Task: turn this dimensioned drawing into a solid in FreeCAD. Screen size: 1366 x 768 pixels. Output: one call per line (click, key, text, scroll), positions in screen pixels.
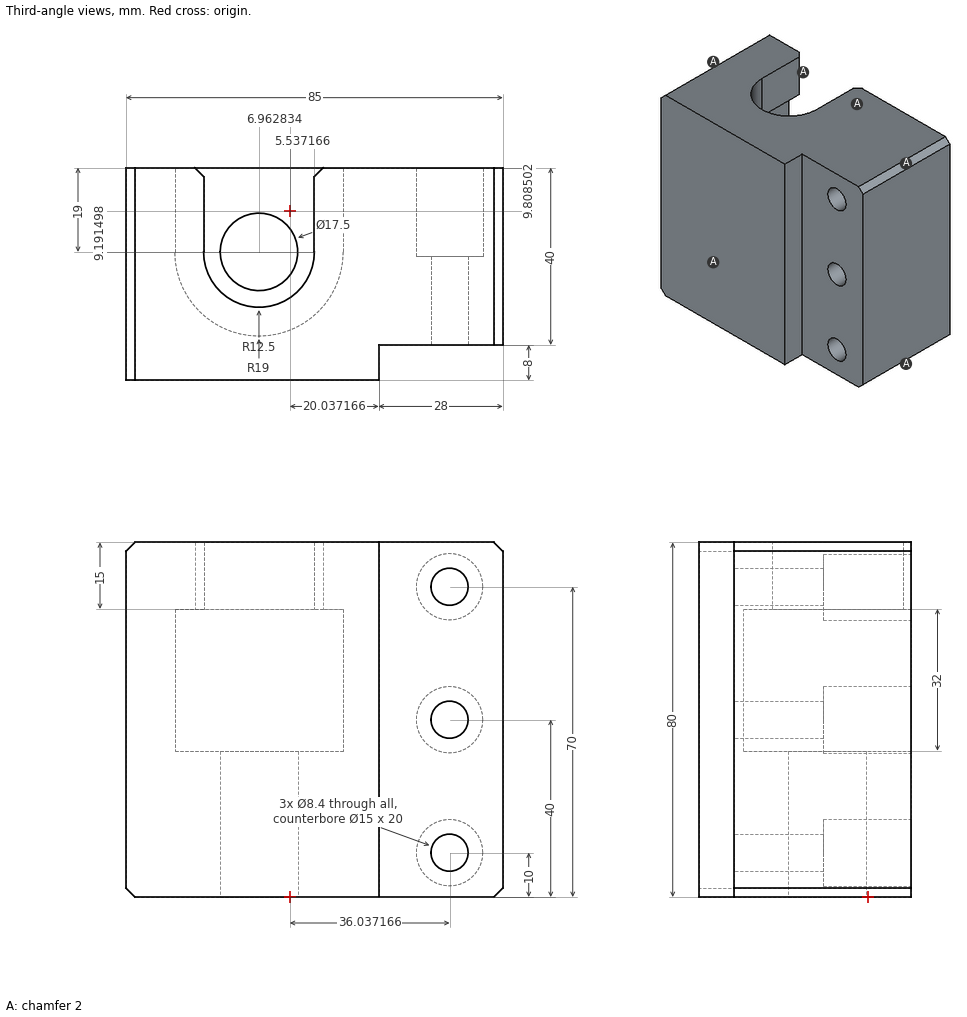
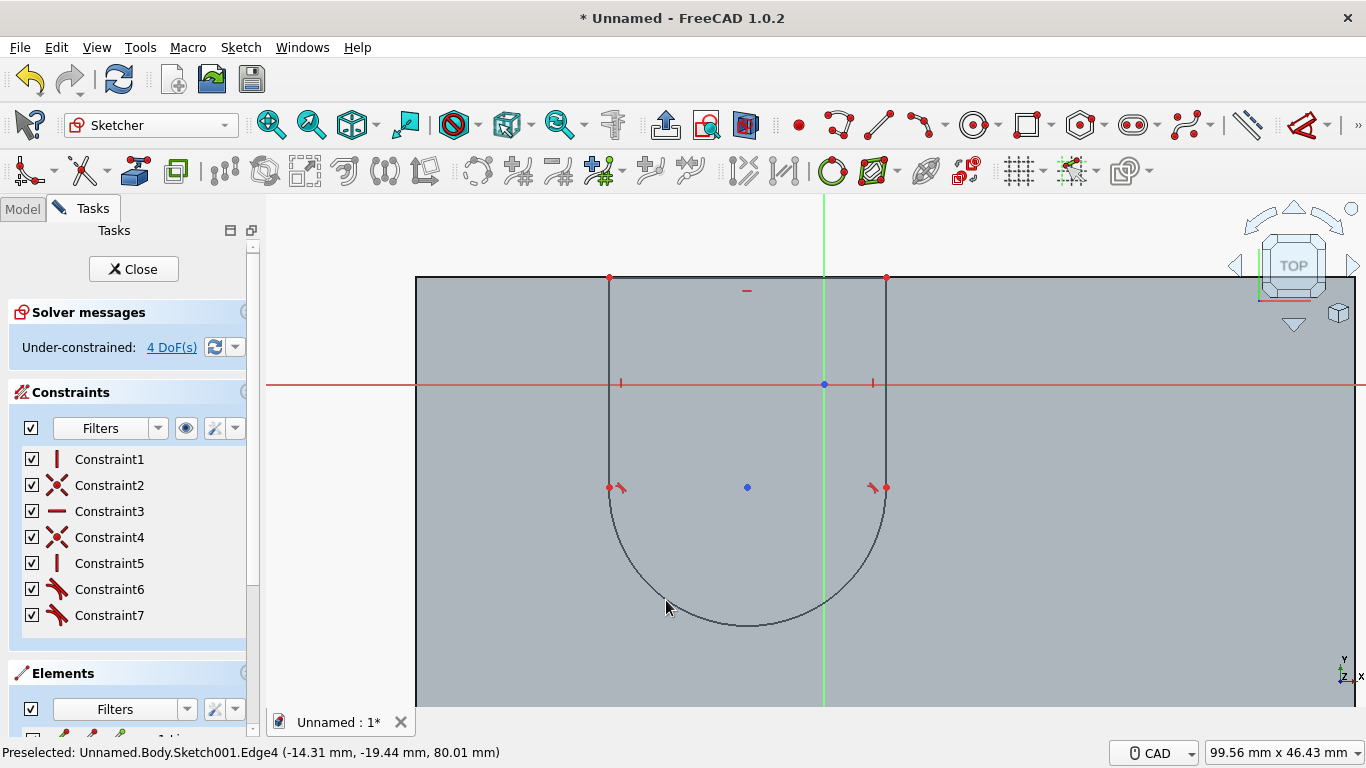
click(1302, 126)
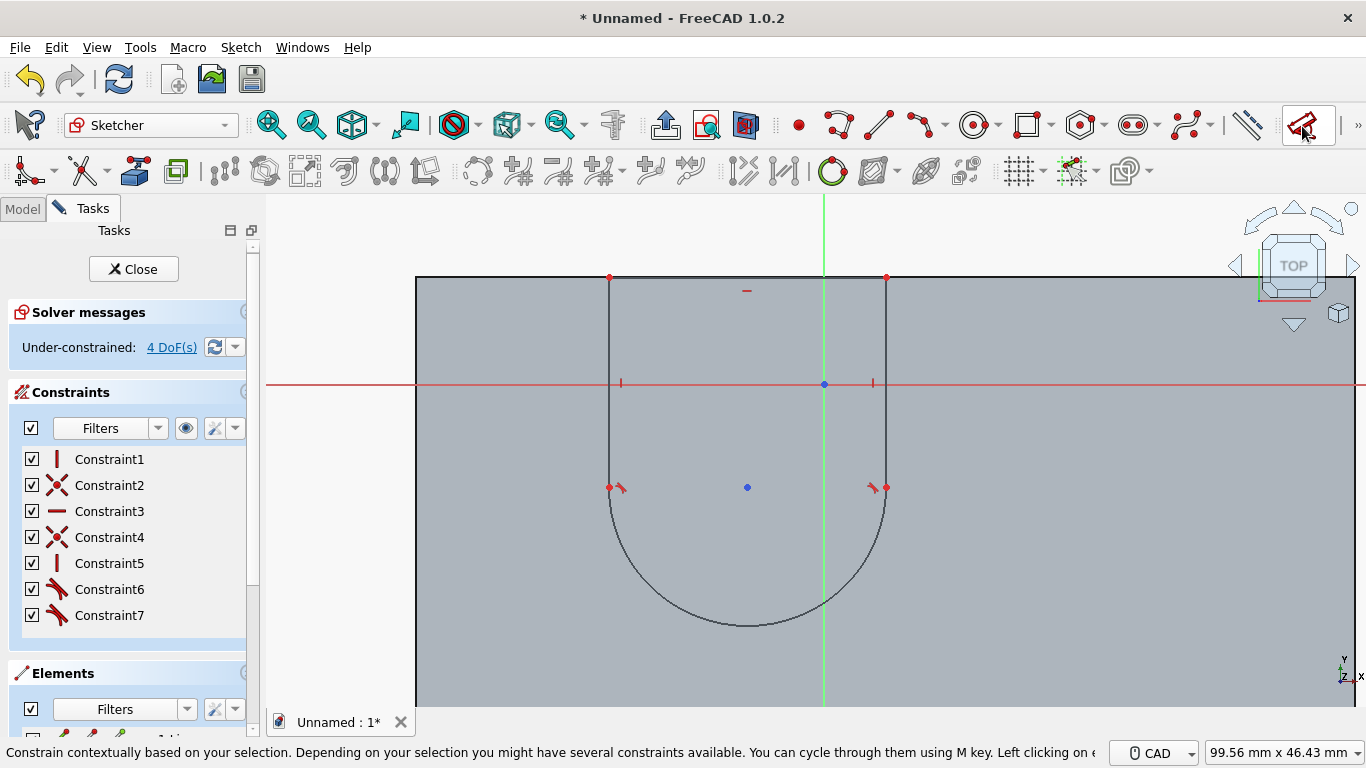
click(666, 600)
click(647, 626)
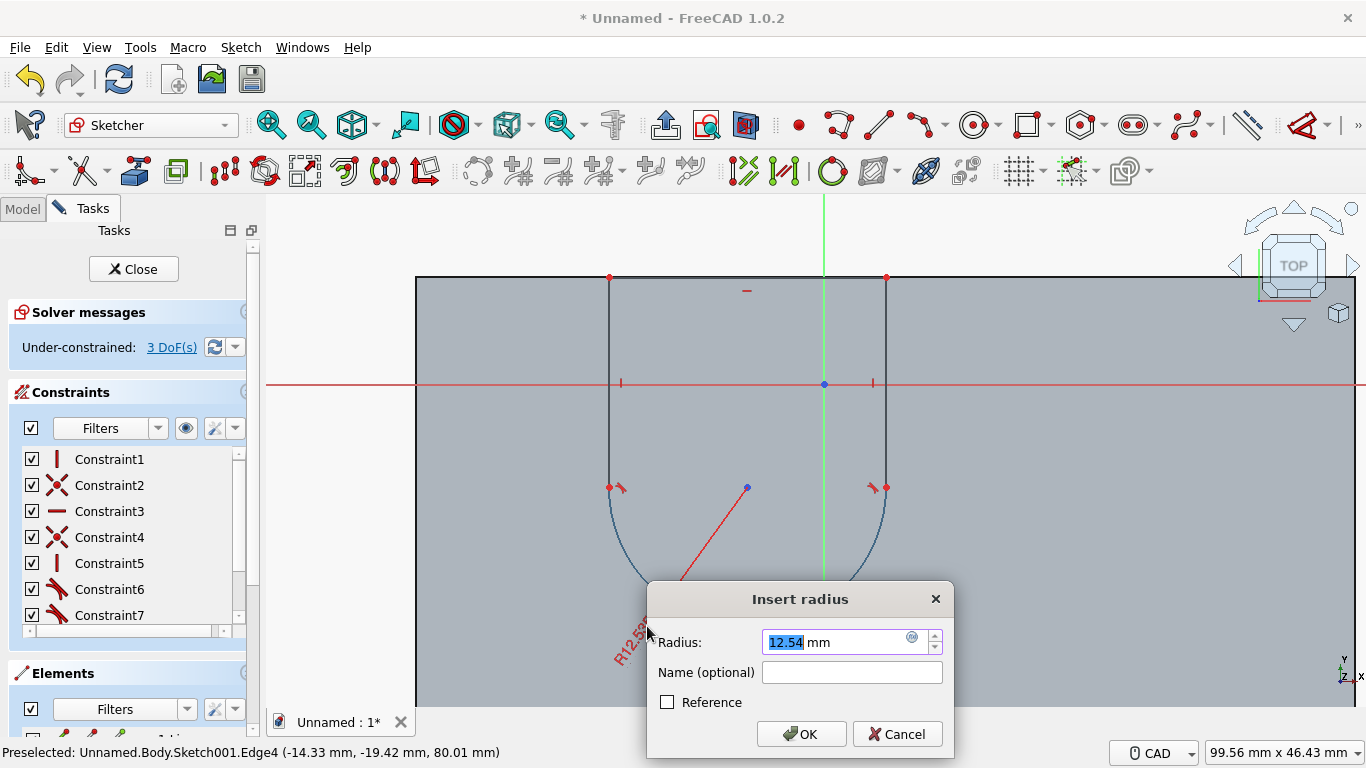
text(12.5)
key(Return)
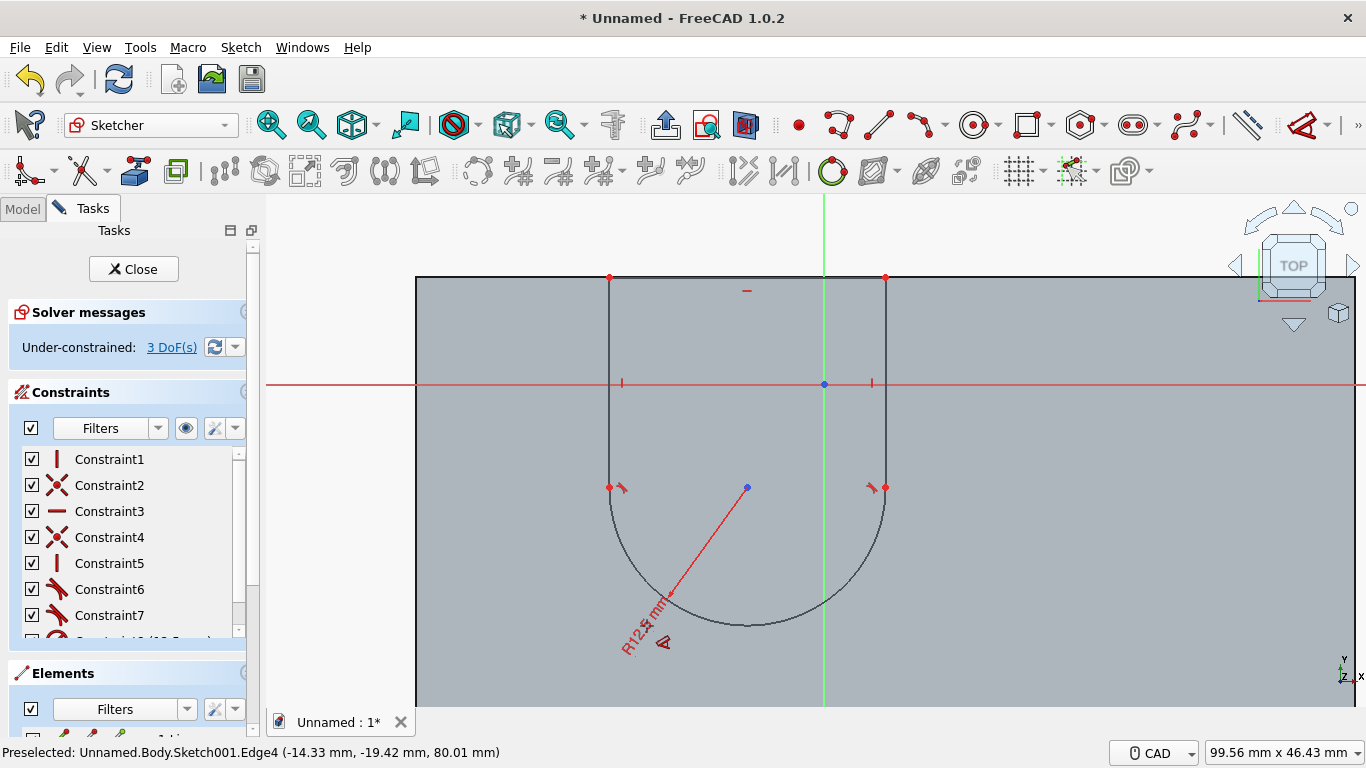
click(886, 425)
click(920, 335)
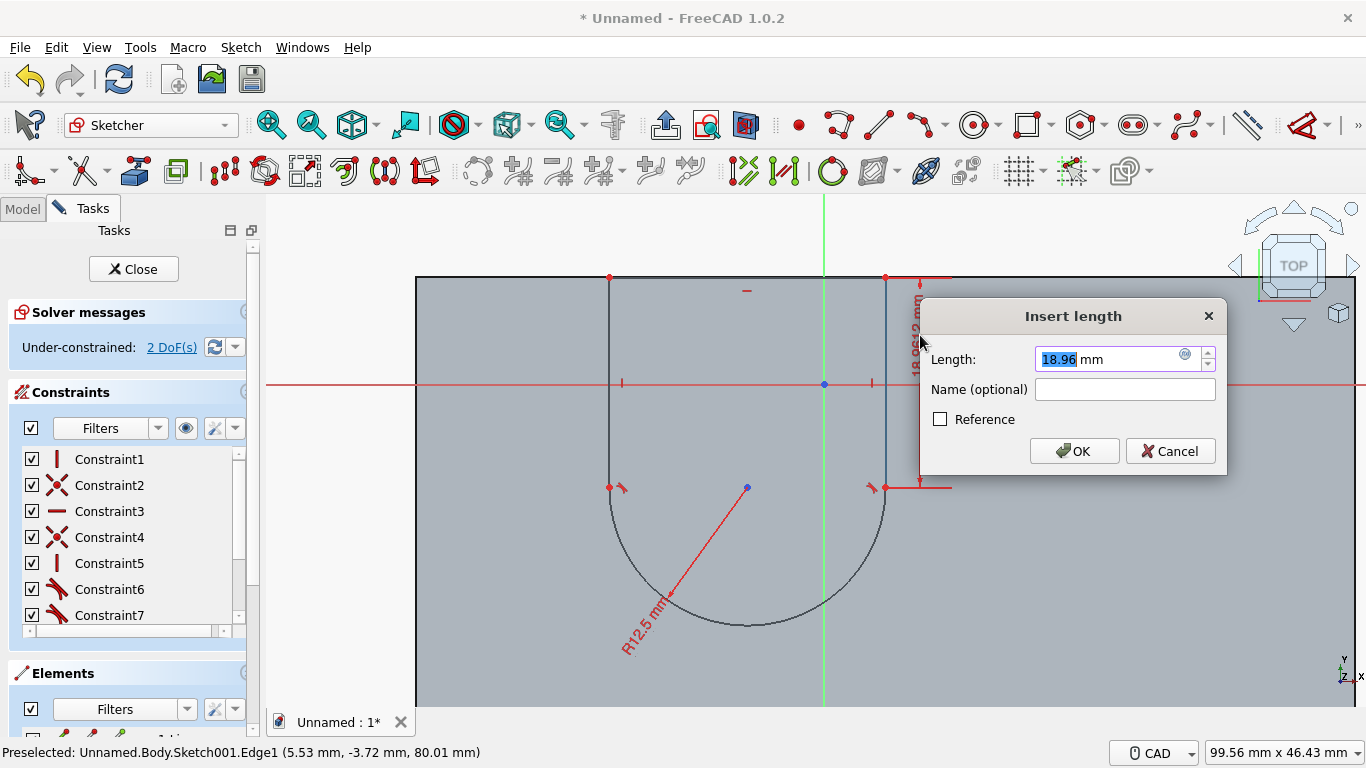
text(19)
key(Return)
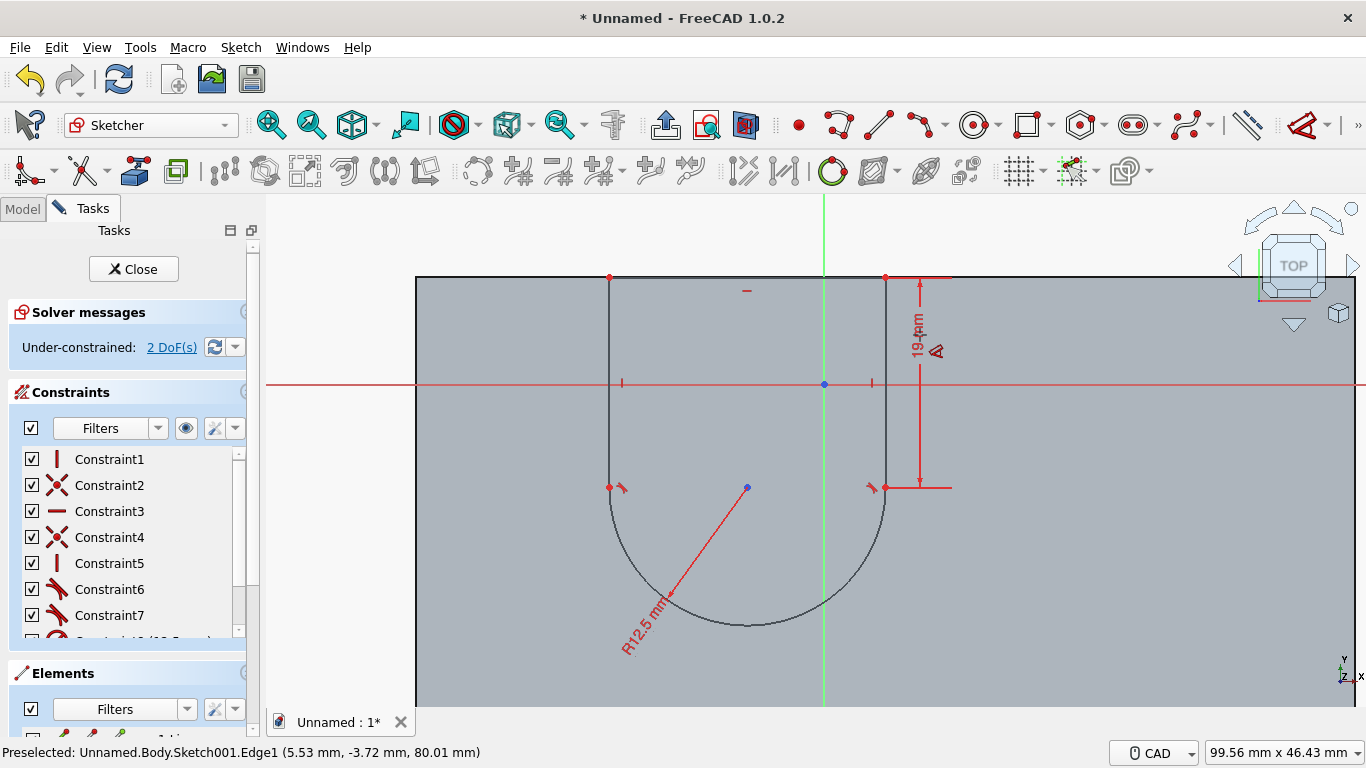
click(886, 488)
click(841, 351)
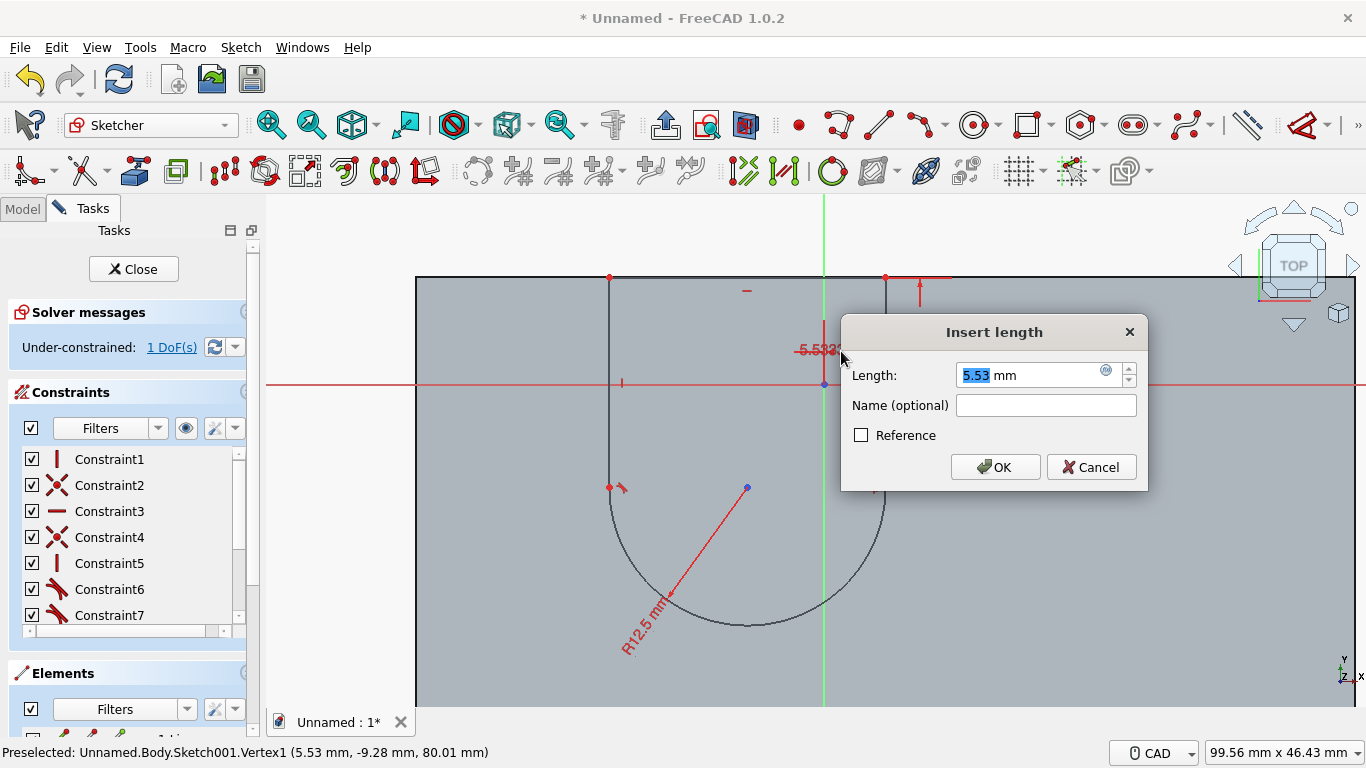
text(5.537166)
key(Return)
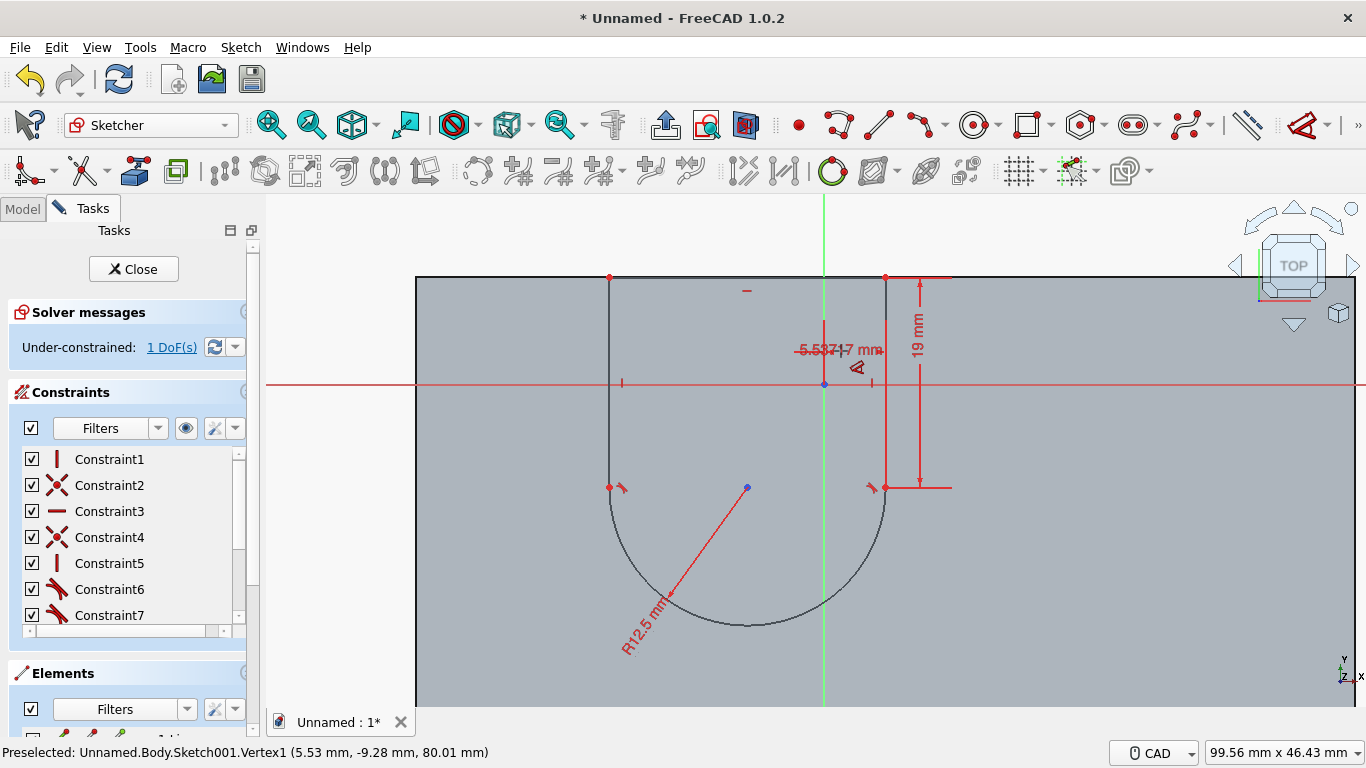
click(886, 488)
click(920, 436)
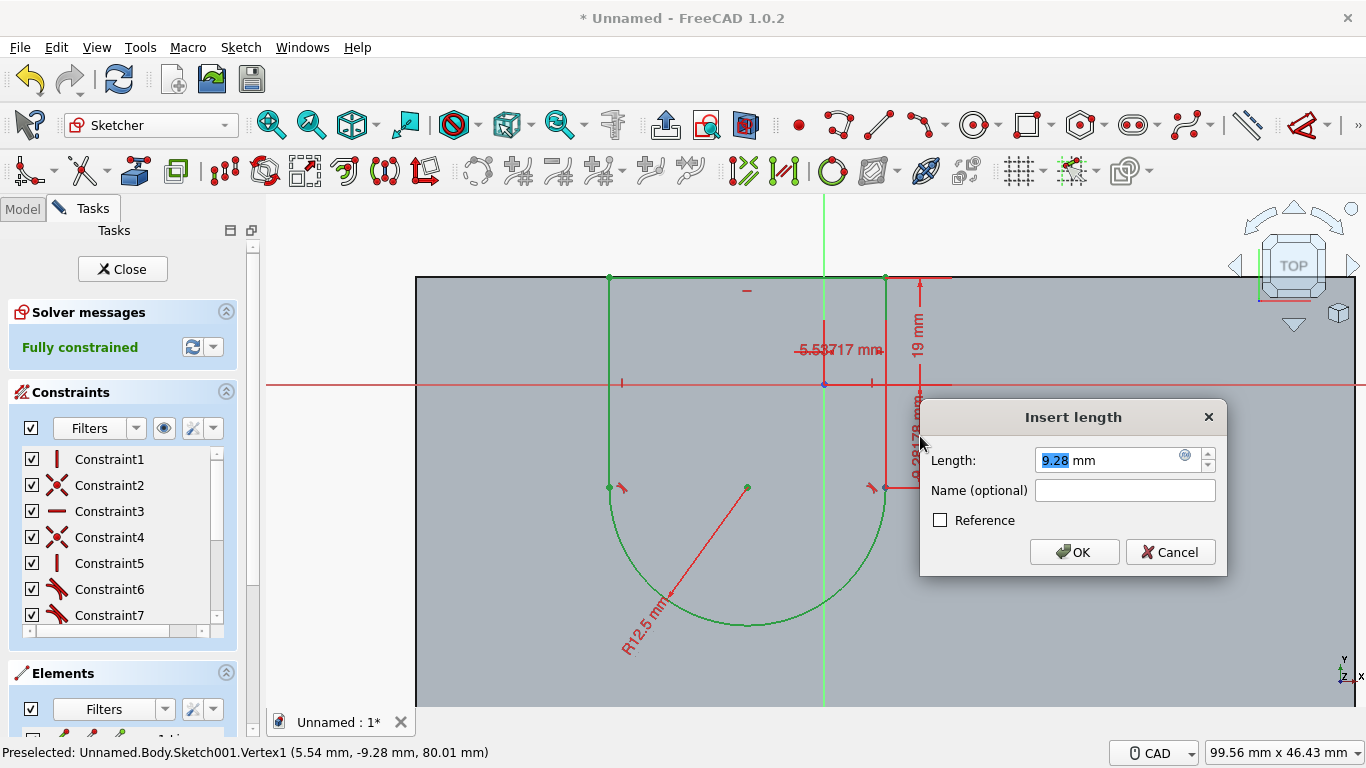
text(9.191498)
key(Return)
key(Escape)